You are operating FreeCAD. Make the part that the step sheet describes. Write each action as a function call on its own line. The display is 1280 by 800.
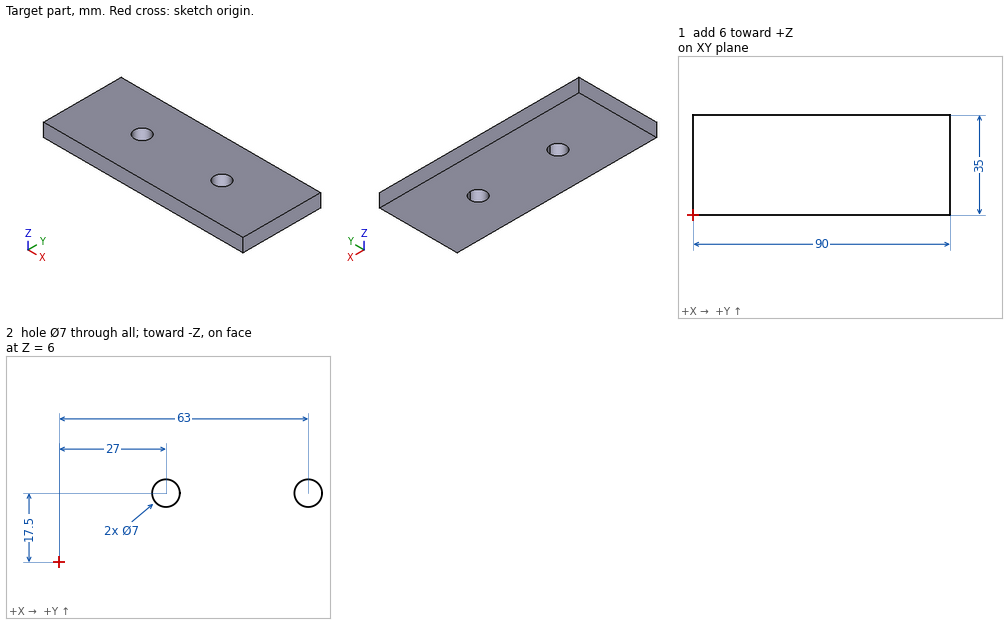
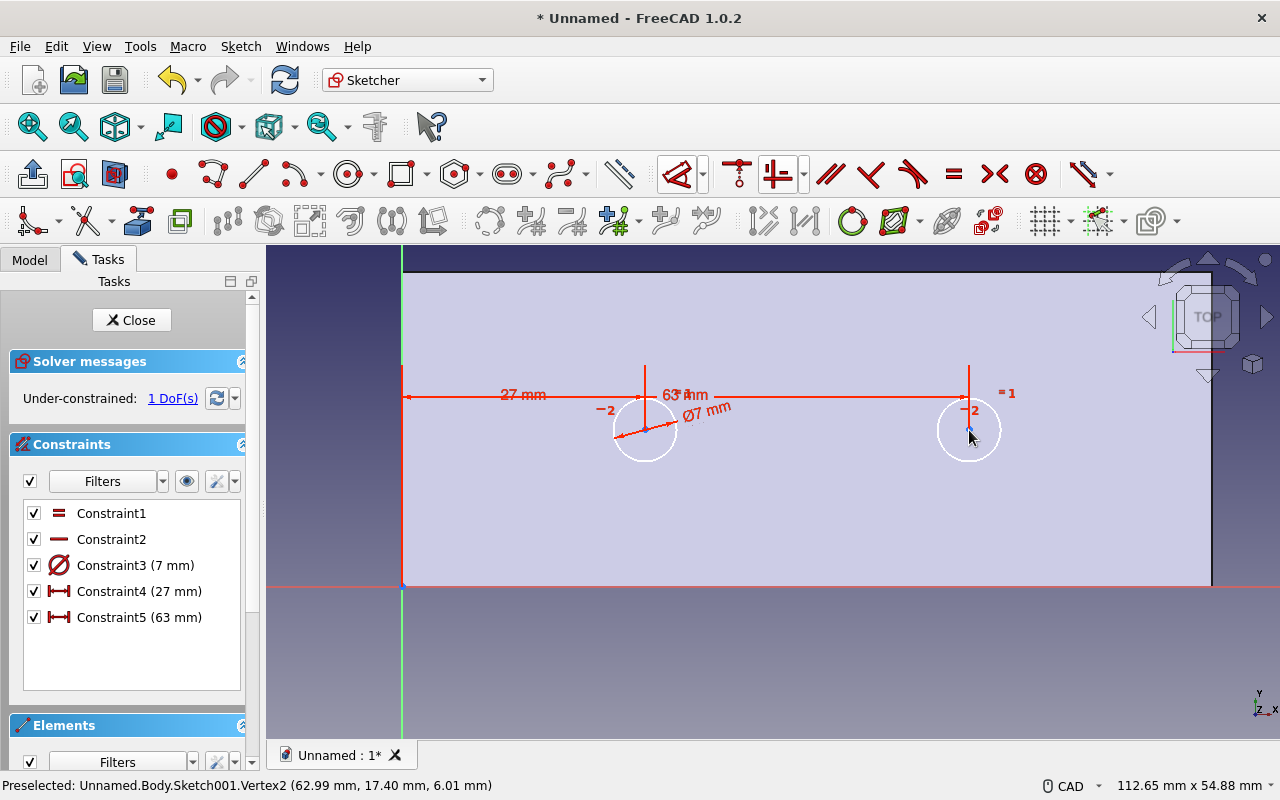
click(645, 430)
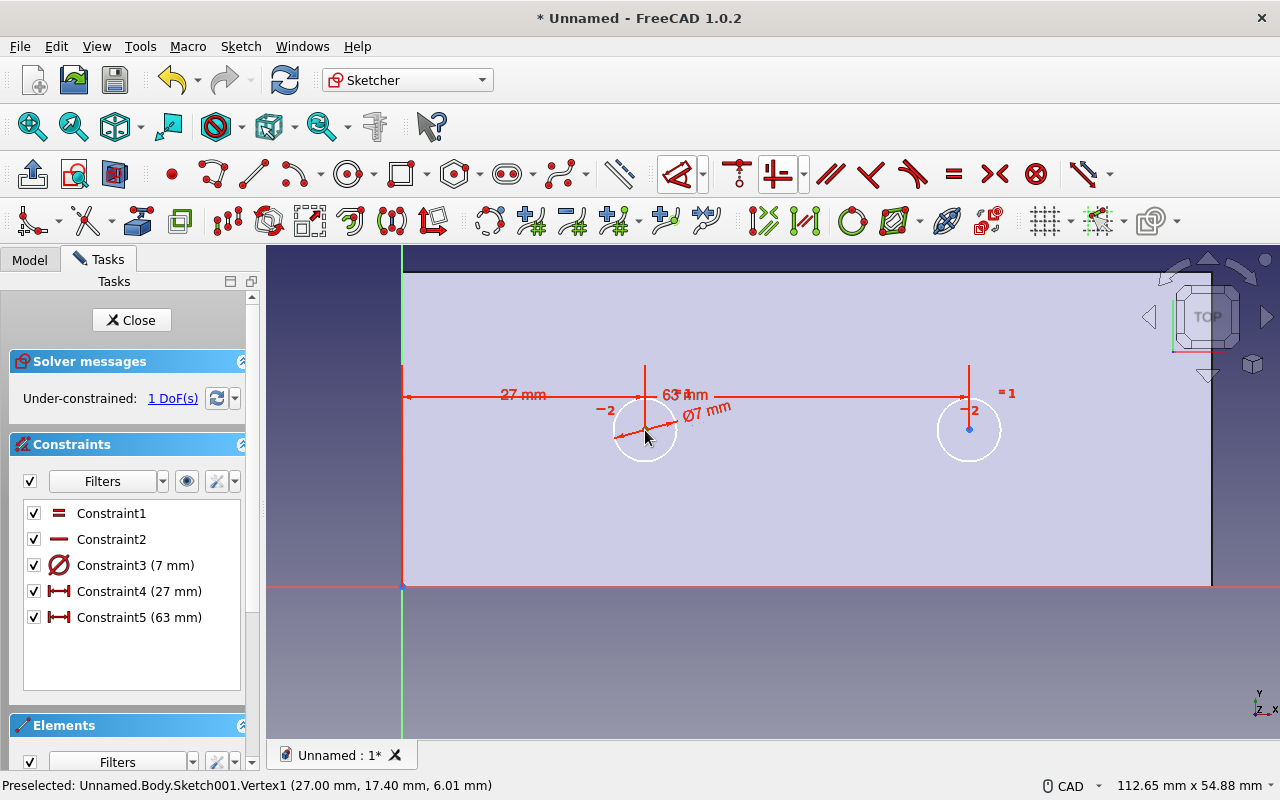
key(i)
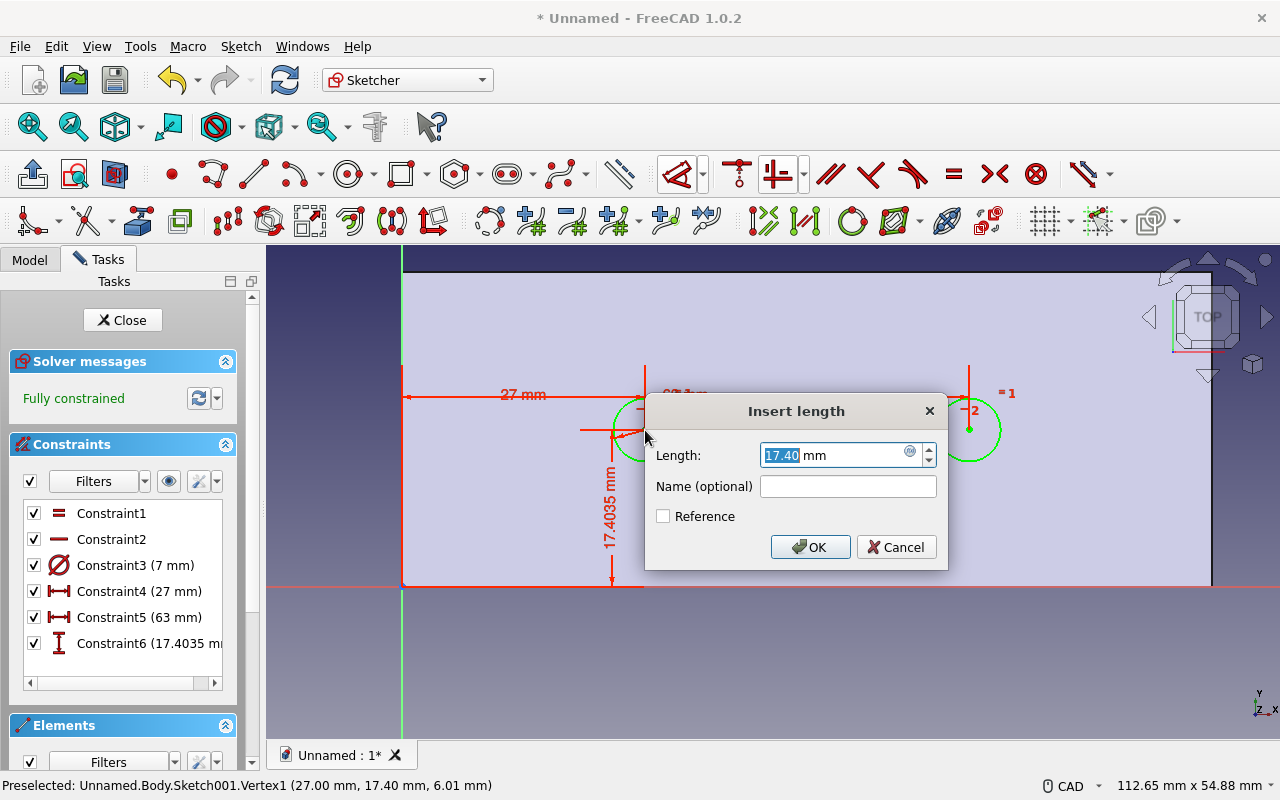
text(17.5)
key(Return)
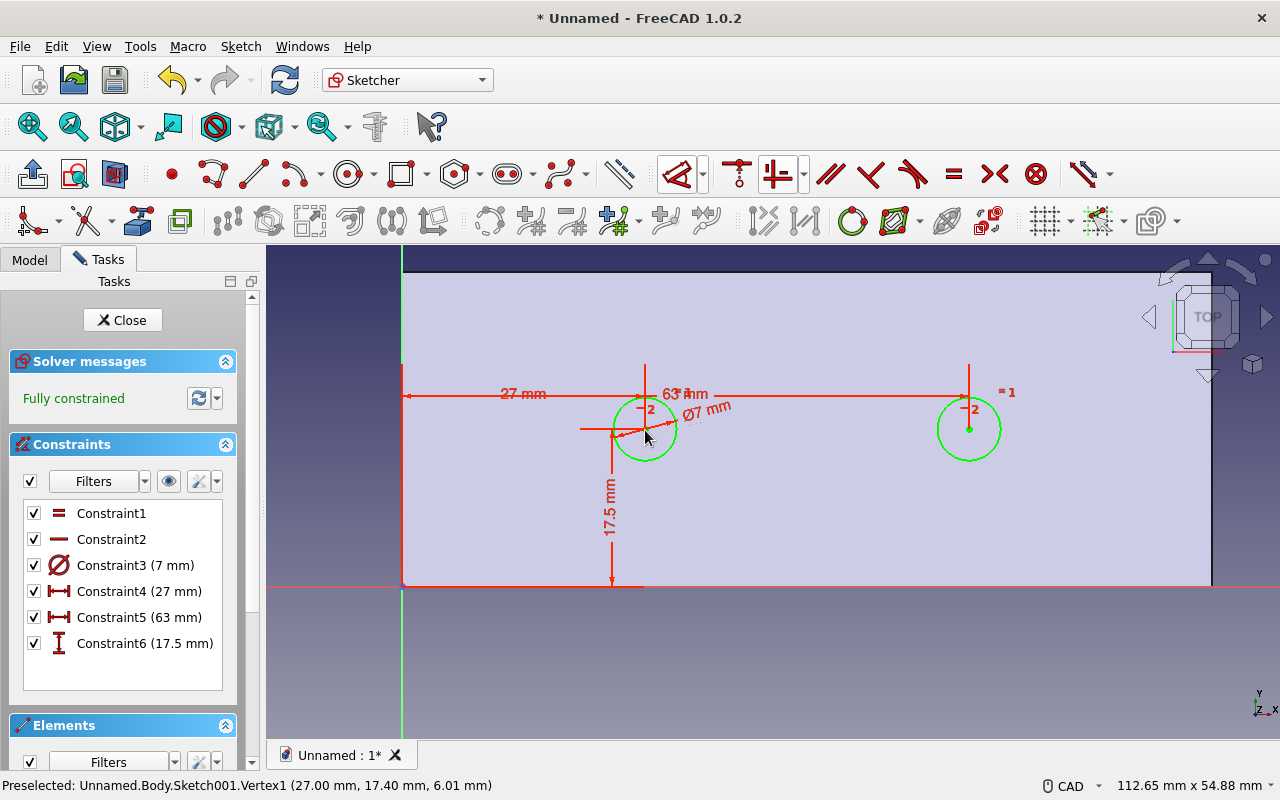
click(123, 320)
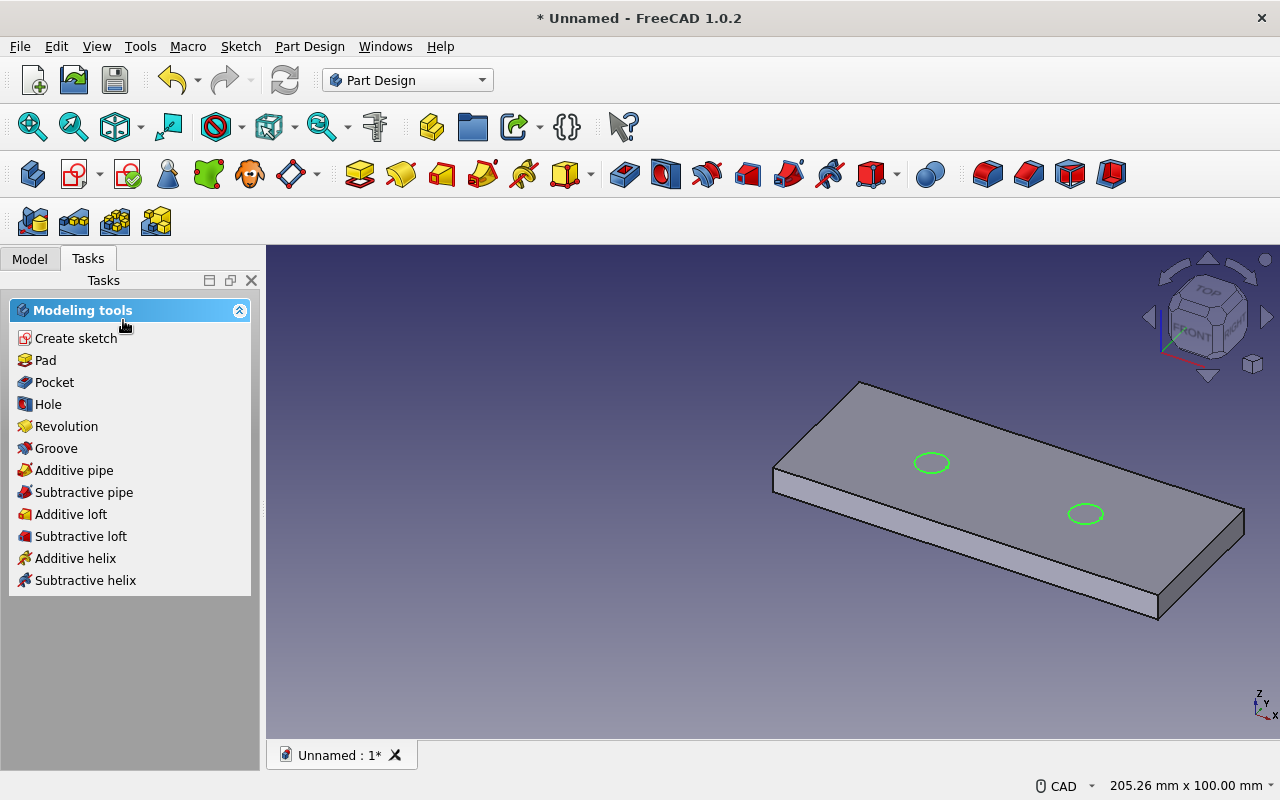
click(666, 174)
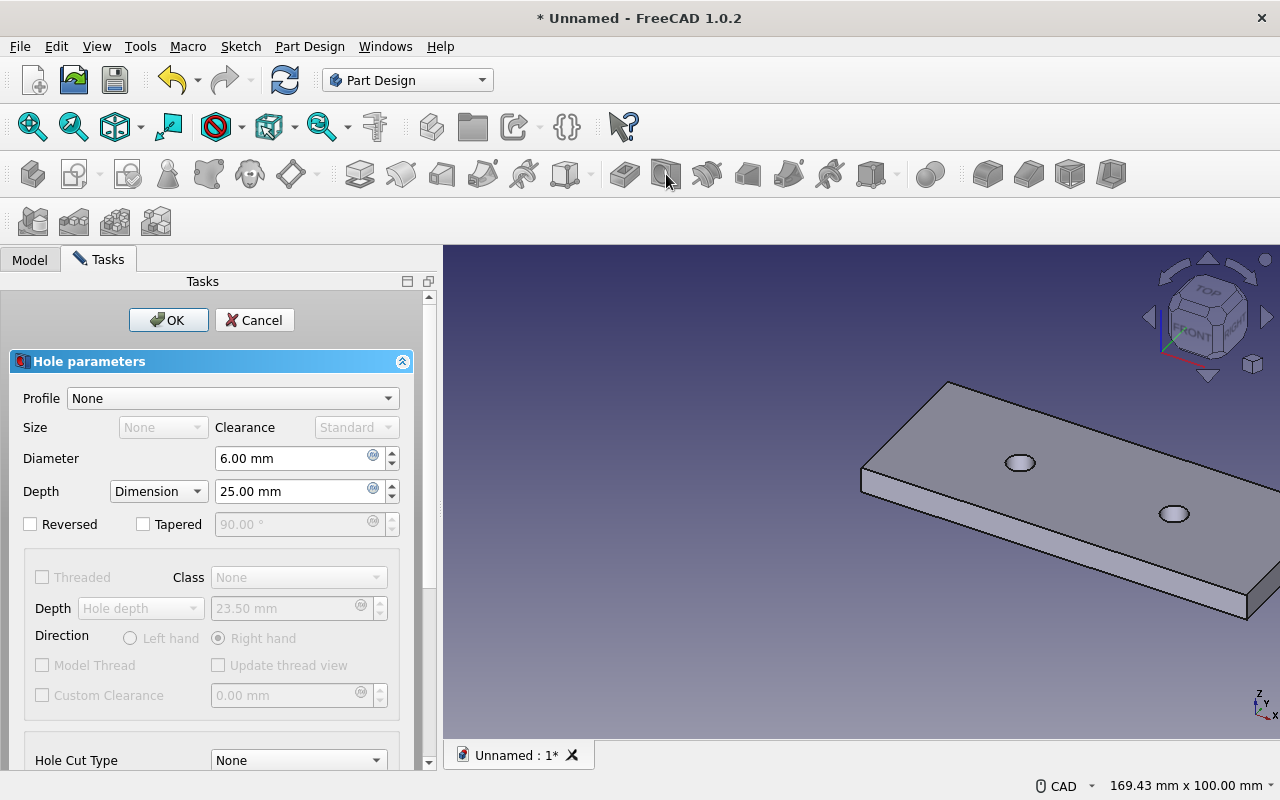
triple_click(300, 458)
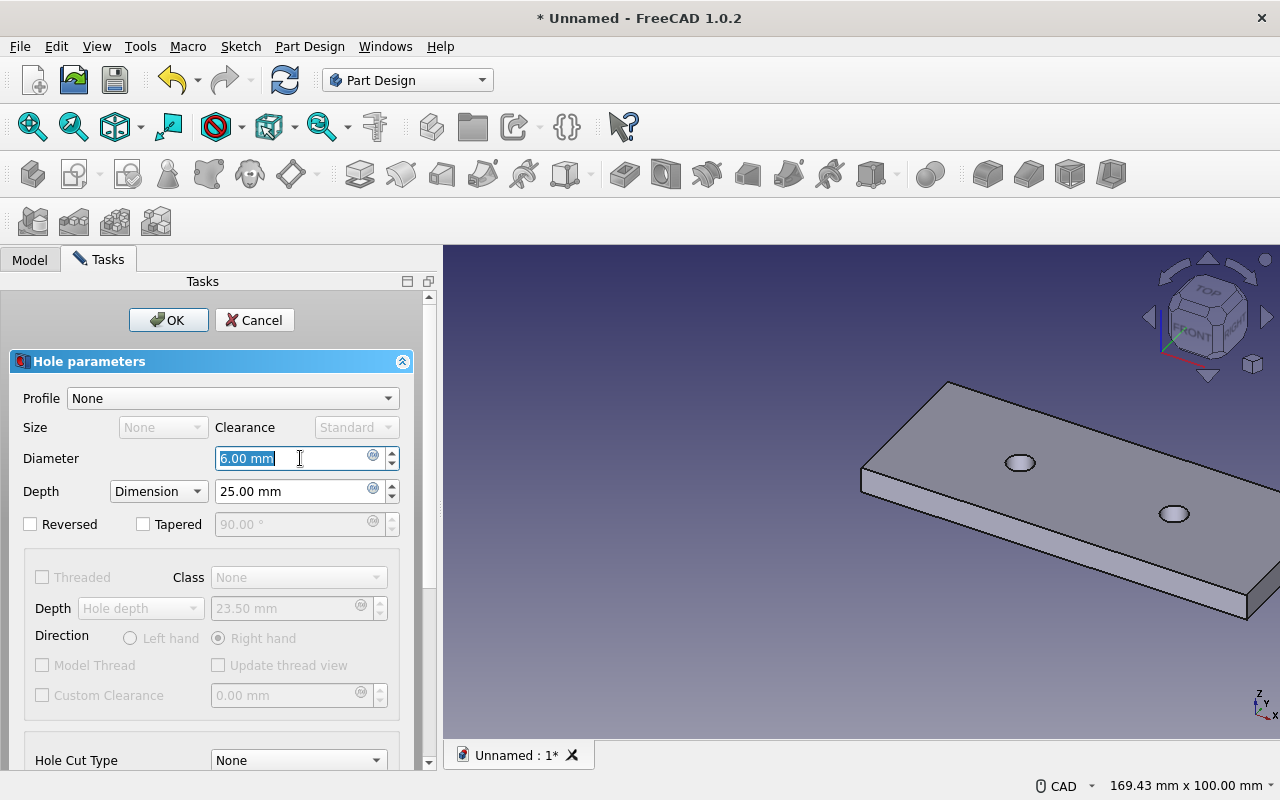
text(7)
key(Tab)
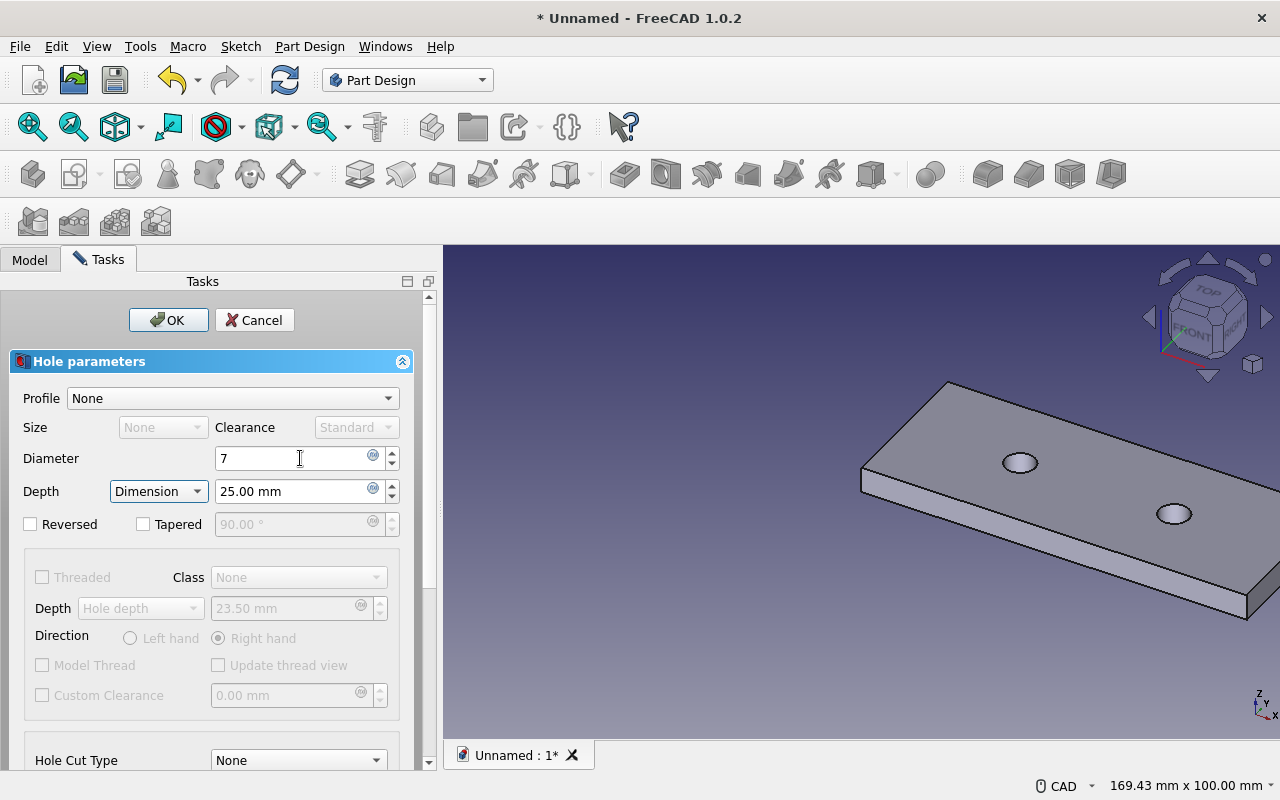
click(160, 492)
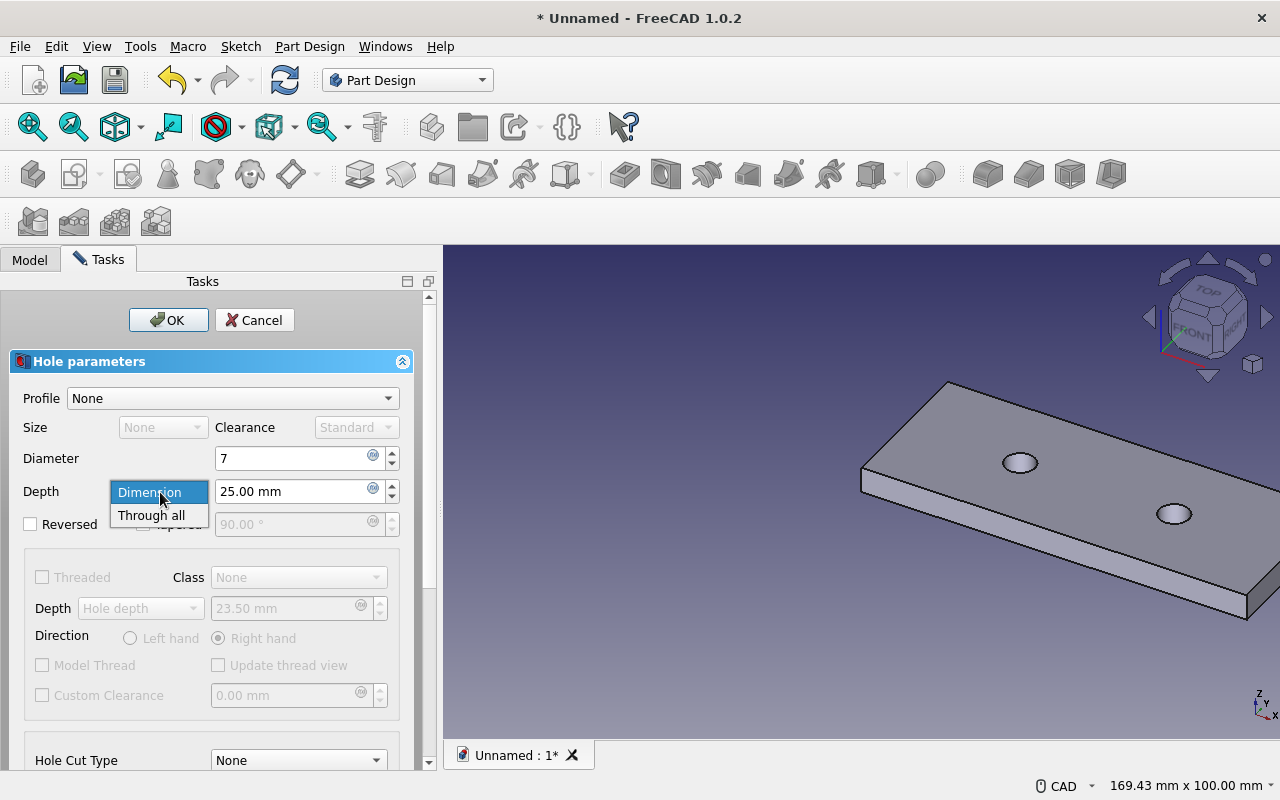
click(158, 516)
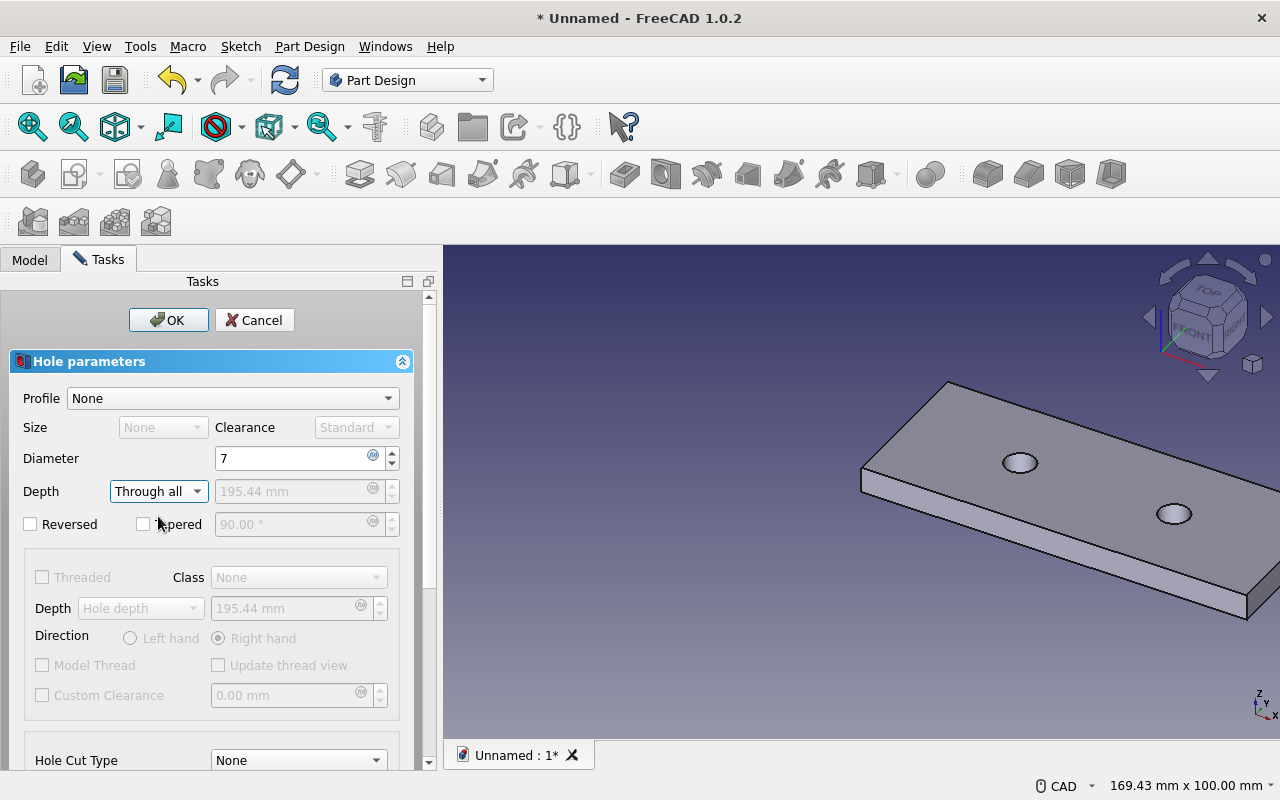
click(169, 320)